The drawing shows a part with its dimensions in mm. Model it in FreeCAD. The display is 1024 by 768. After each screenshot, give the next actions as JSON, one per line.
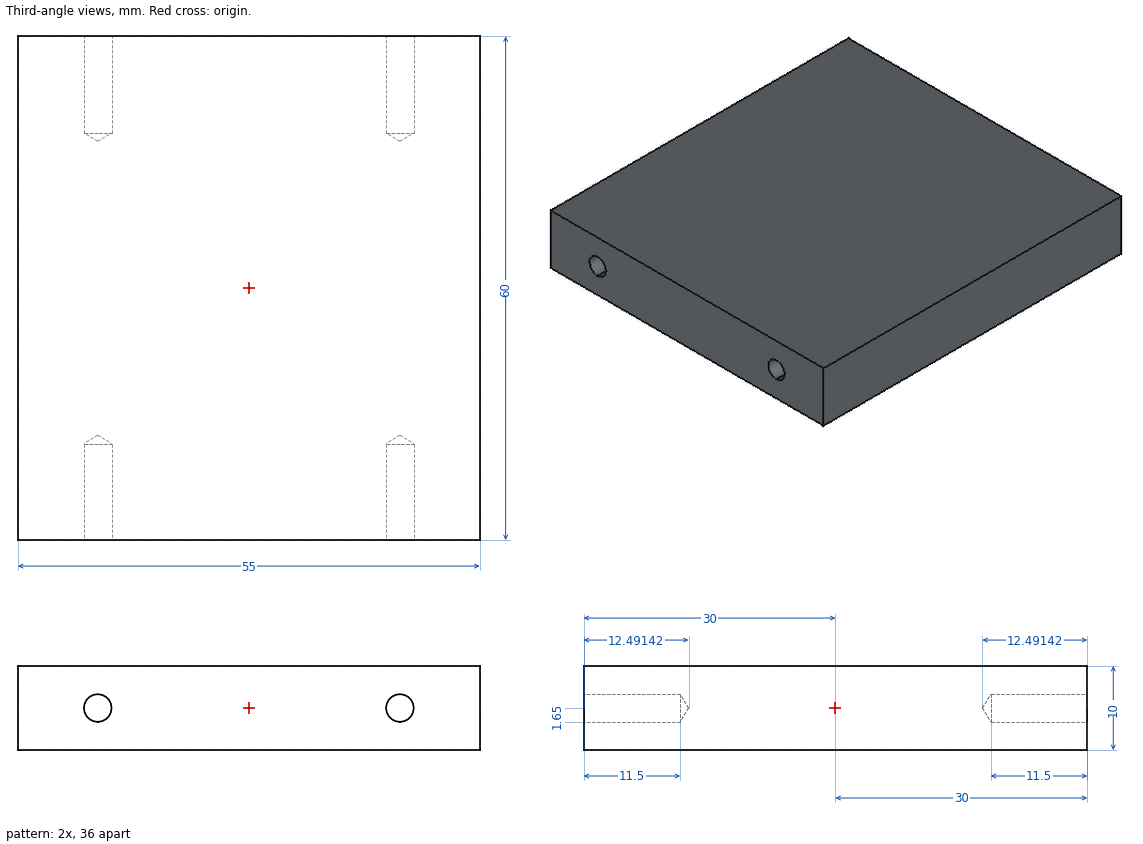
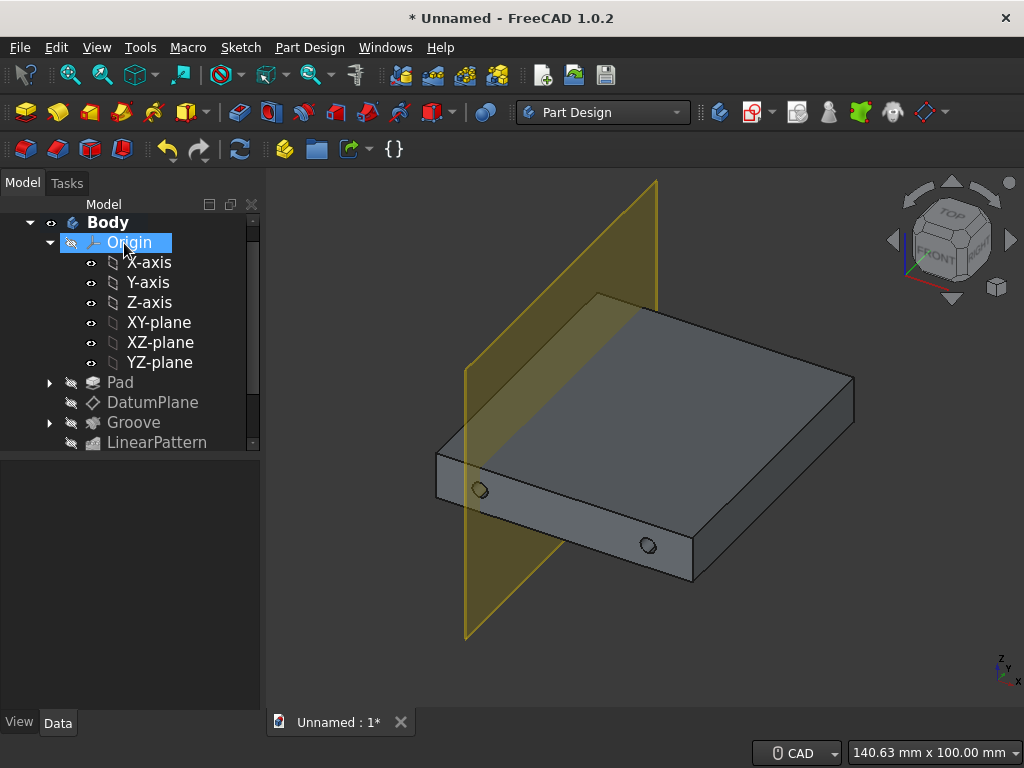
{"action": "scroll", "coordinate": [120, 338], "scroll_direction": "down", "scroll_amount": 3}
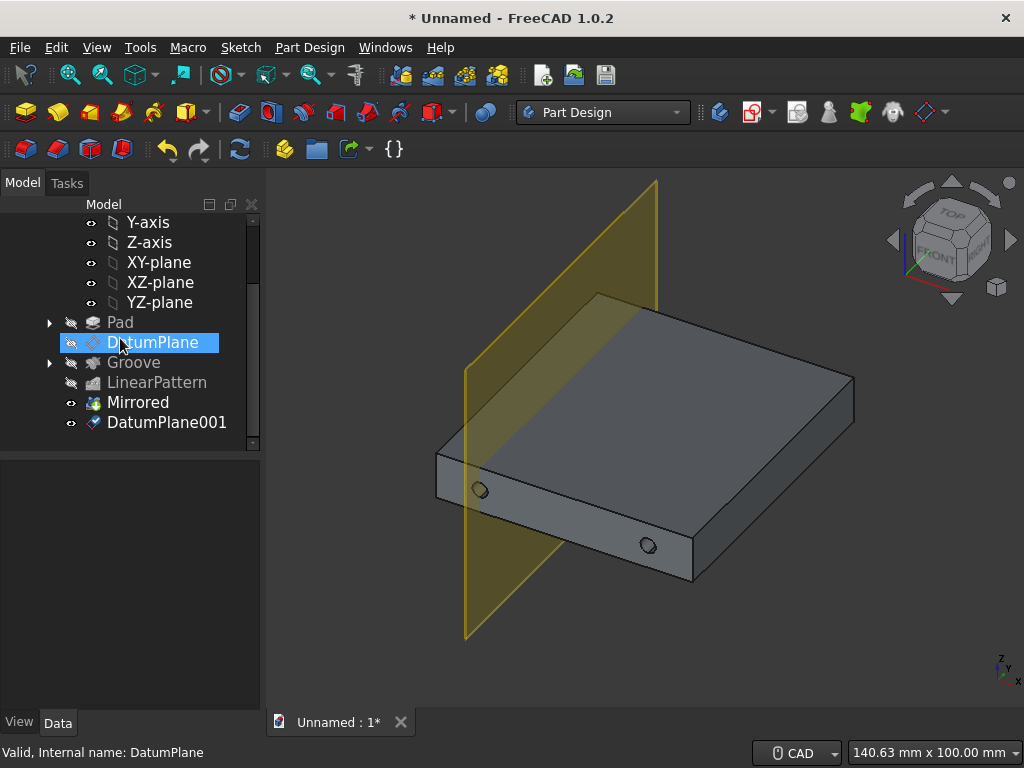
{"action": "left_click", "coordinate": [116, 423]}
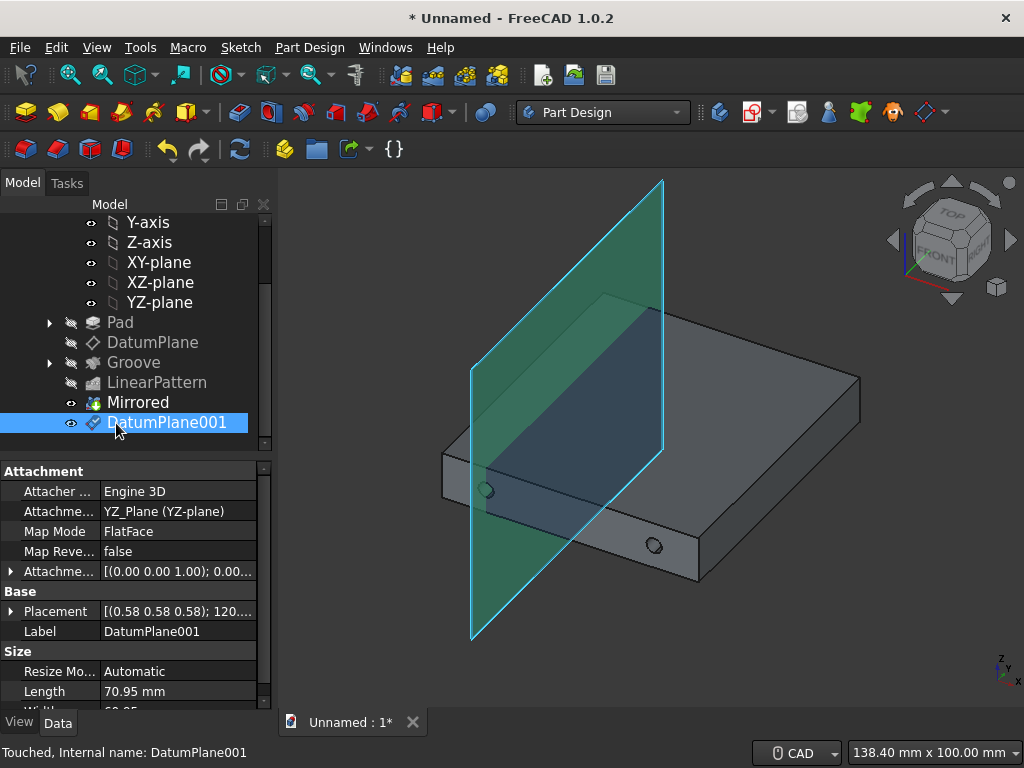
{"action": "left_click", "coordinate": [752, 112]}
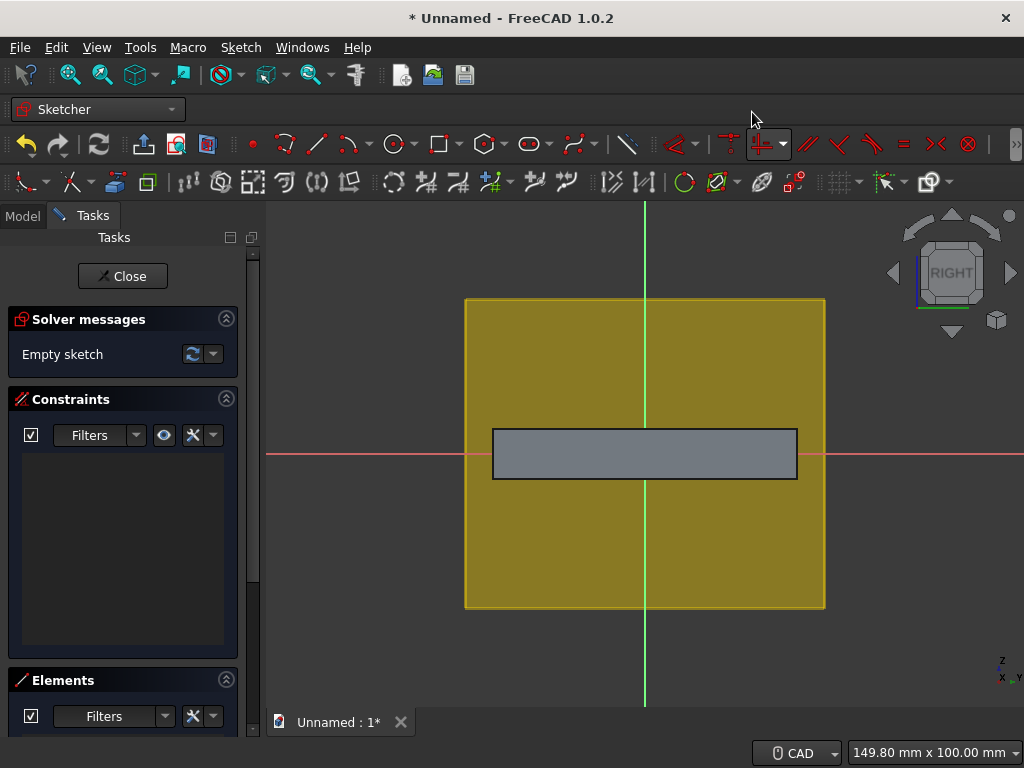
{"action": "left_click", "coordinate": [208, 144]}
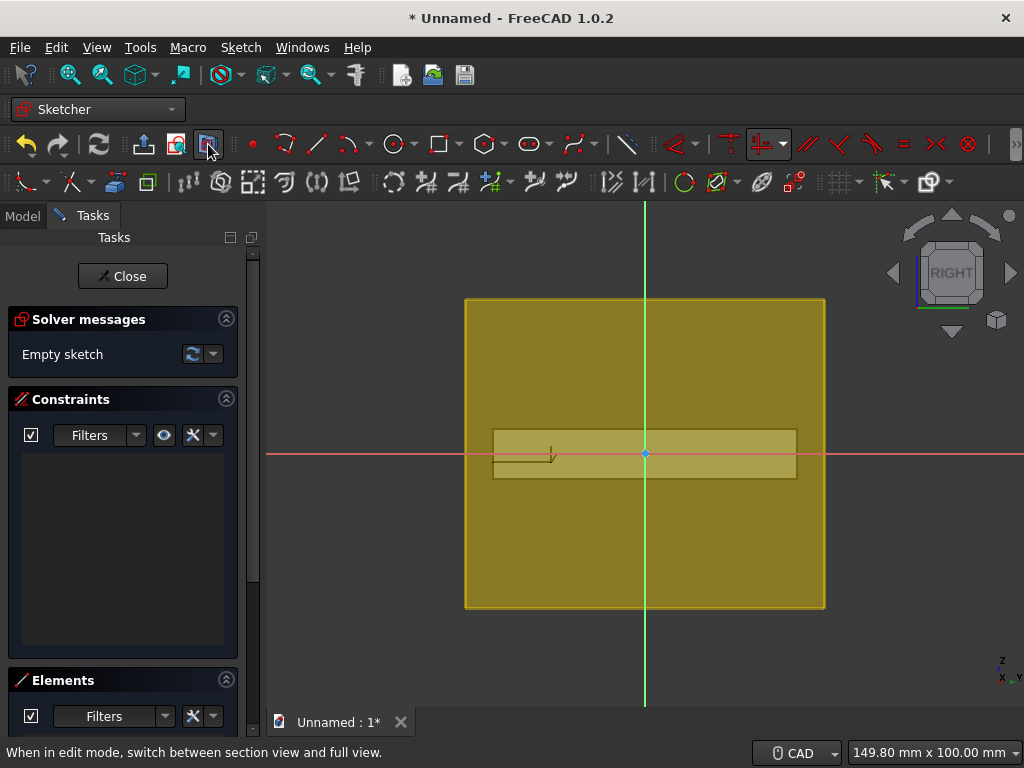
{"action": "scroll", "coordinate": [805, 461], "scroll_direction": "up", "scroll_amount": 5}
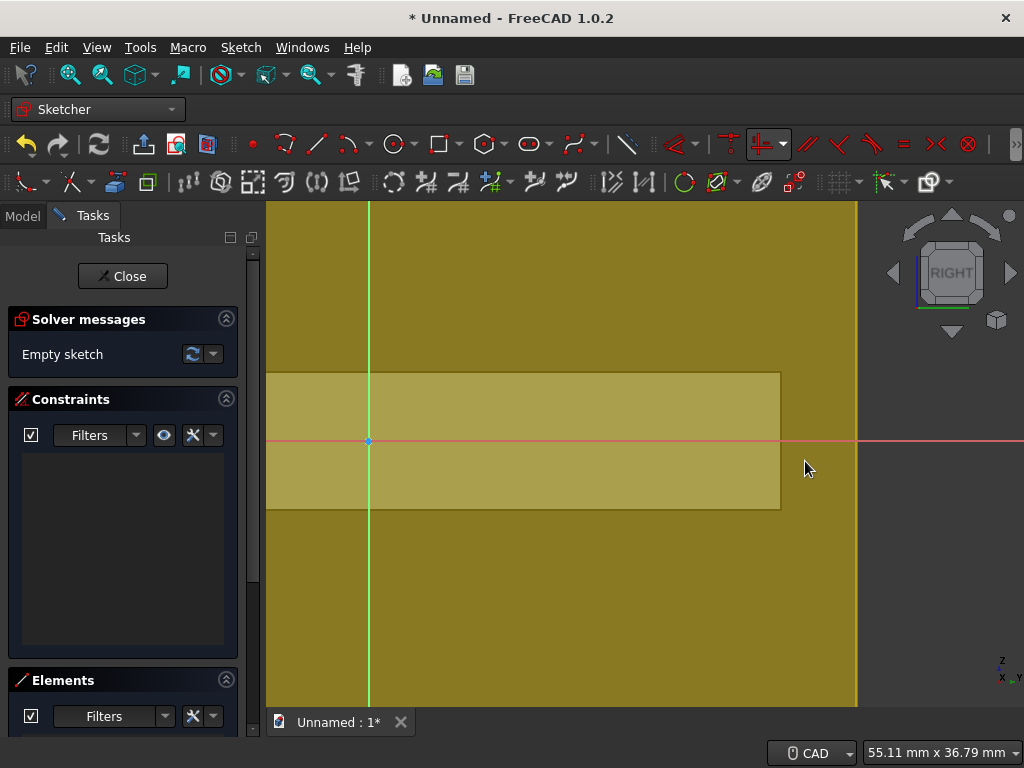
{"action": "left_click", "coordinate": [286, 144]}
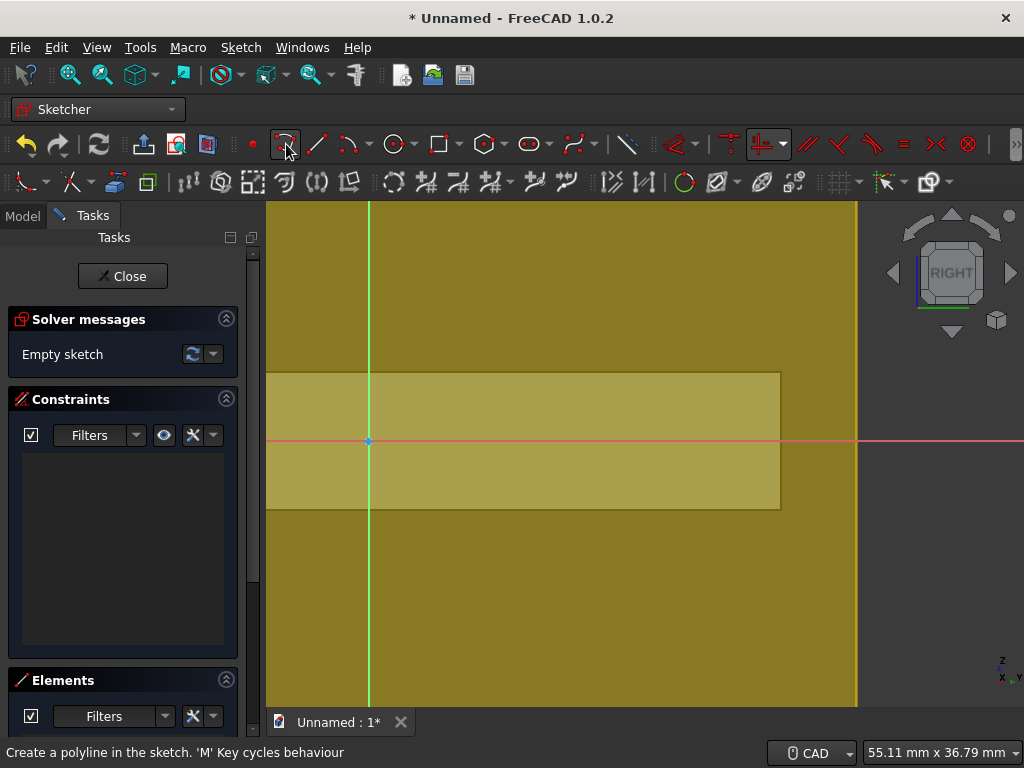
{"action": "left_click", "coordinate": [610, 441]}
{"action": "left_click", "coordinate": [623, 464]}
{"action": "left_click", "coordinate": [781, 464]}
{"action": "left_click", "coordinate": [781, 450]}
{"action": "left_click", "coordinate": [610, 441]}
{"action": "key", "text": "Escape"}
{"action": "key", "text": "Escape"}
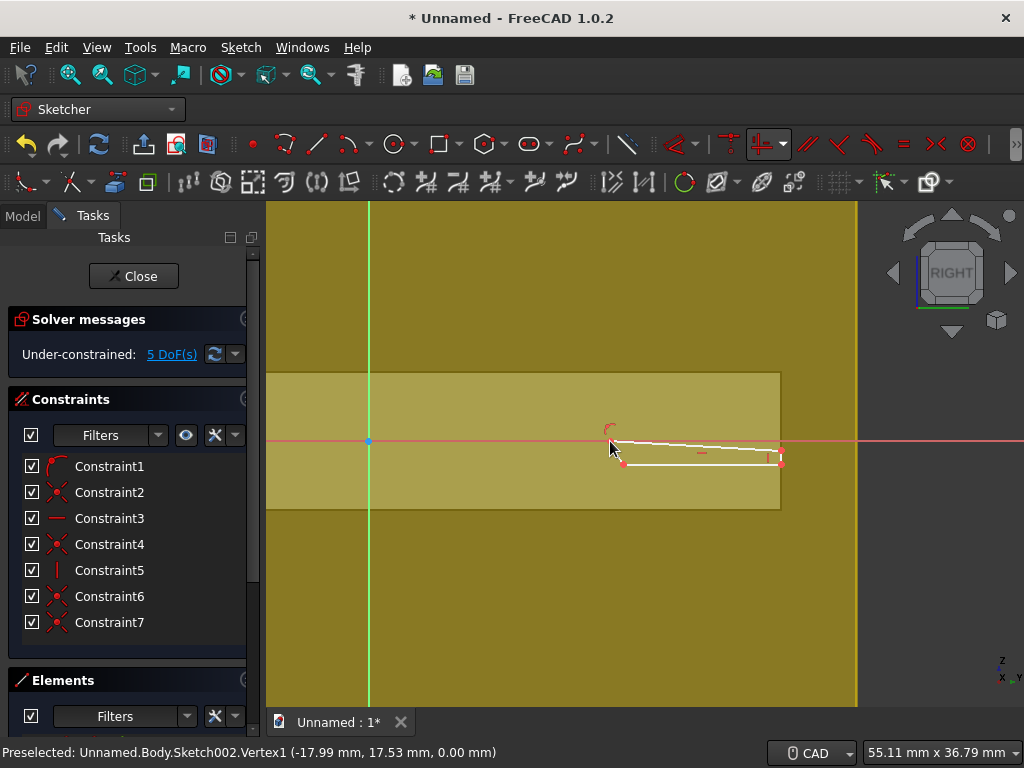
{"action": "left_click", "coordinate": [661, 444]}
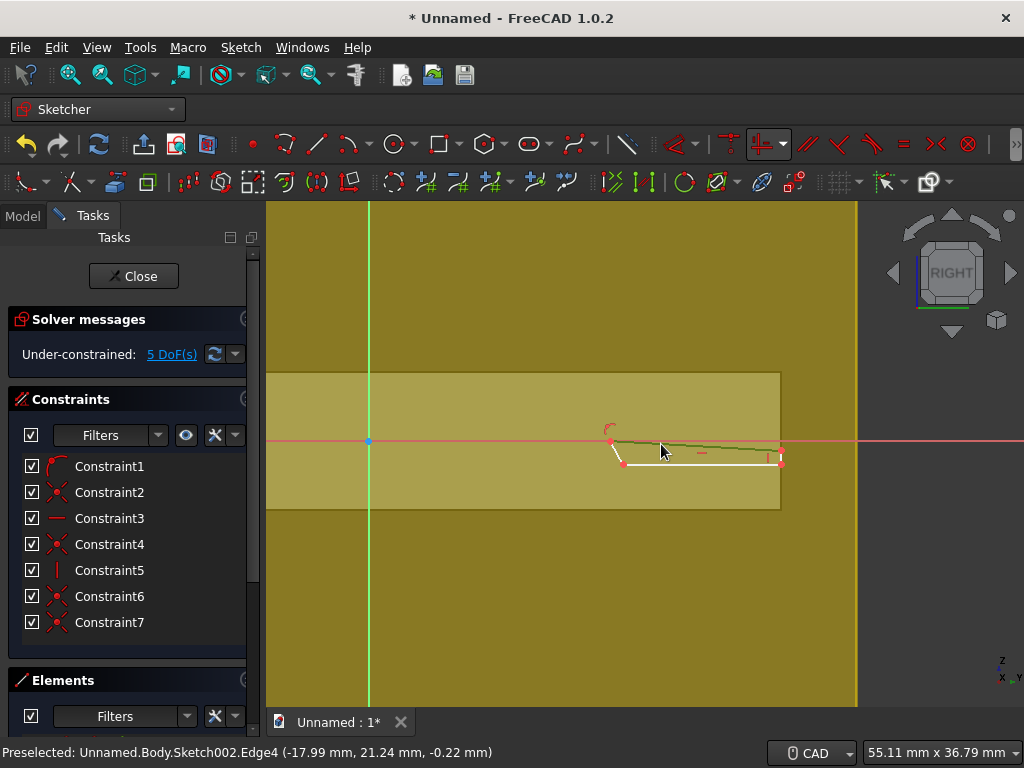
{"action": "key", "text": "h"}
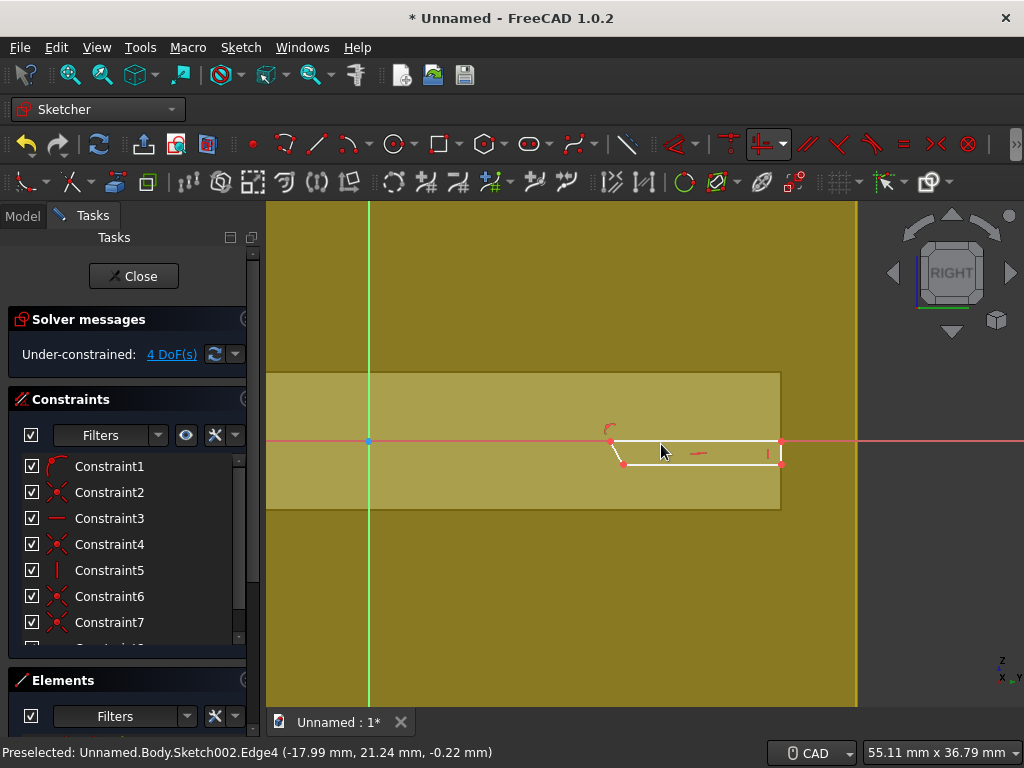
{"action": "left_click", "coordinate": [674, 144]}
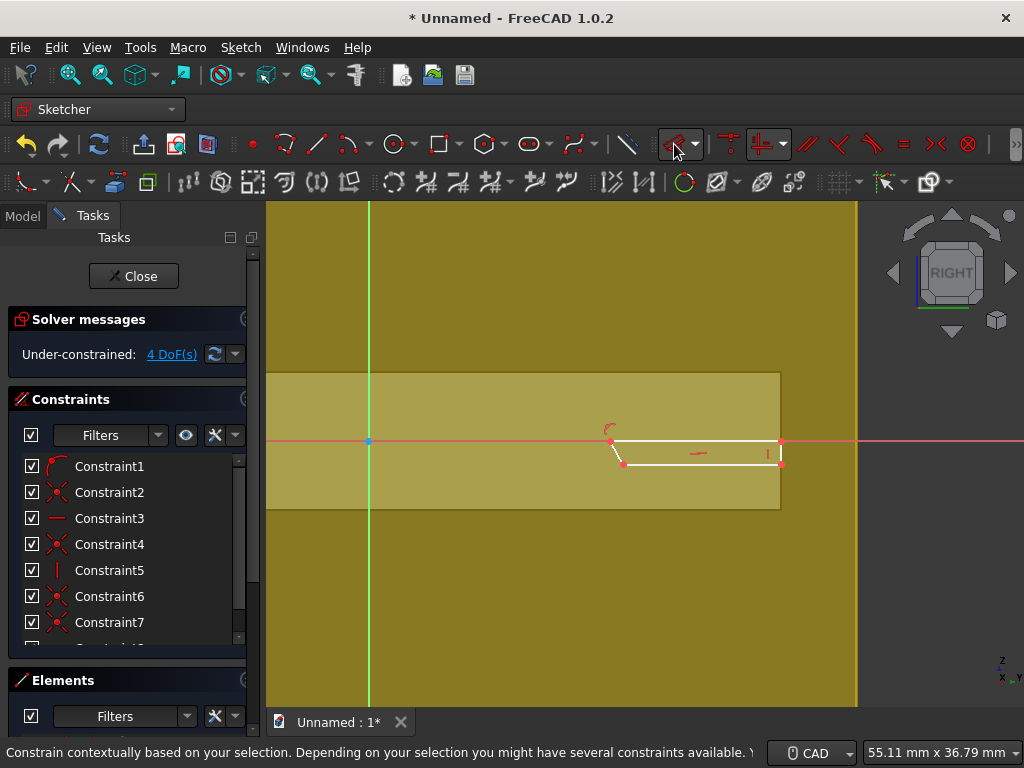
{"action": "left_click", "coordinate": [781, 465]}
{"action": "left_click", "coordinate": [575, 499]}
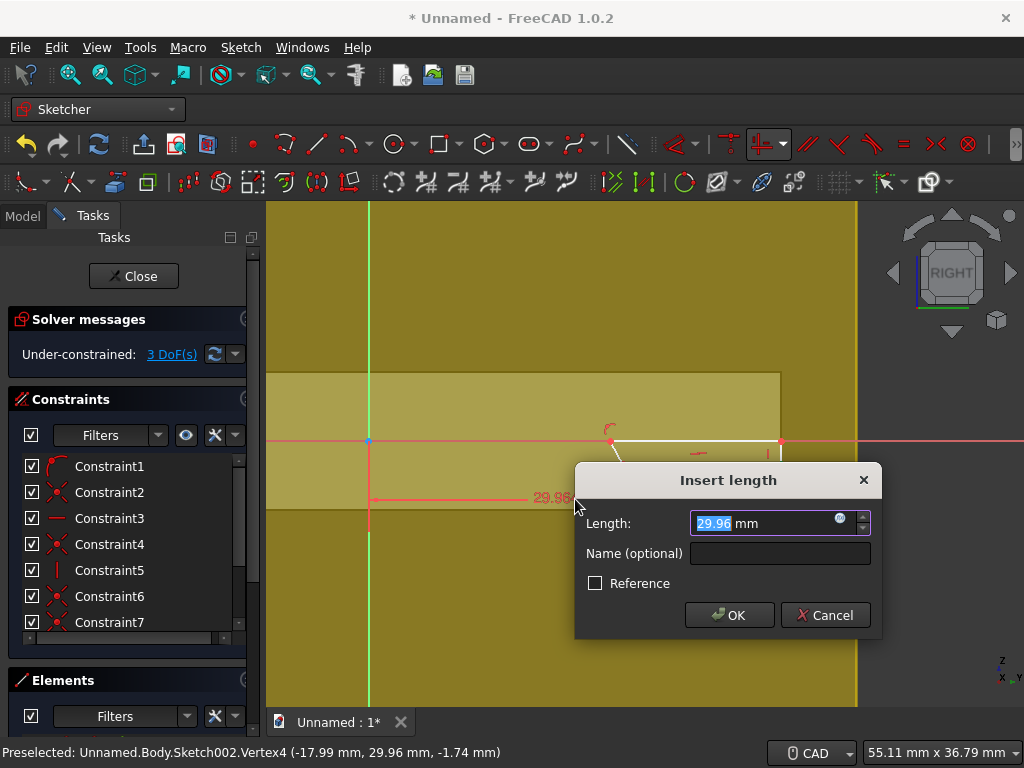
{"action": "type", "text": "30"}
{"action": "key", "text": "Return"}